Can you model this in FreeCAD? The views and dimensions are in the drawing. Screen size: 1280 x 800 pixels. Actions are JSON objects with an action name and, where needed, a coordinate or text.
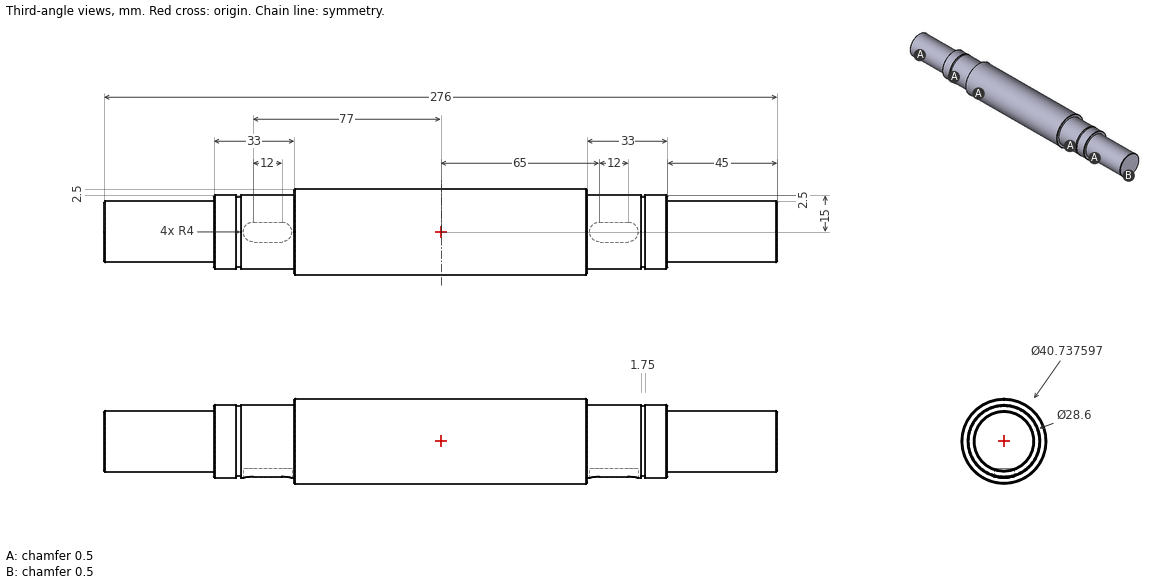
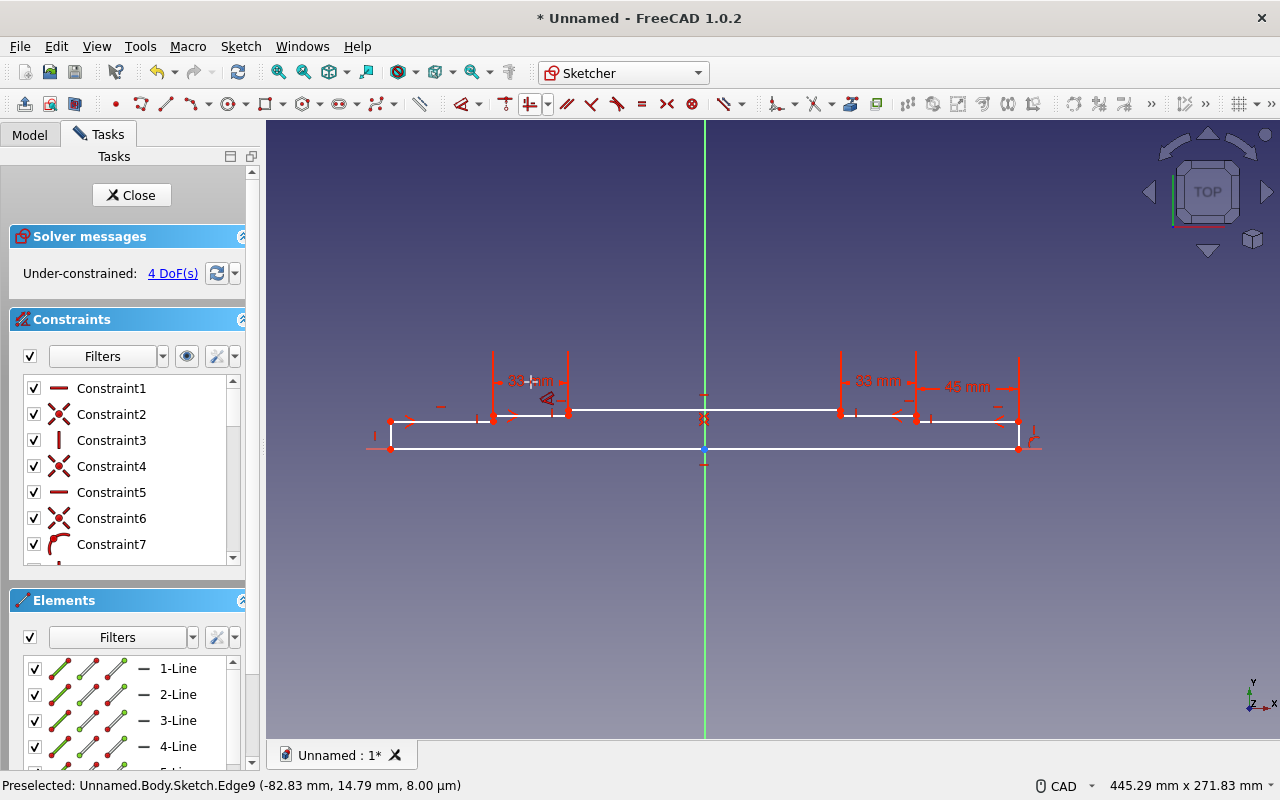
{"action": "scroll", "coordinate": [916, 419], "scroll_direction": "up", "scroll_amount": 10}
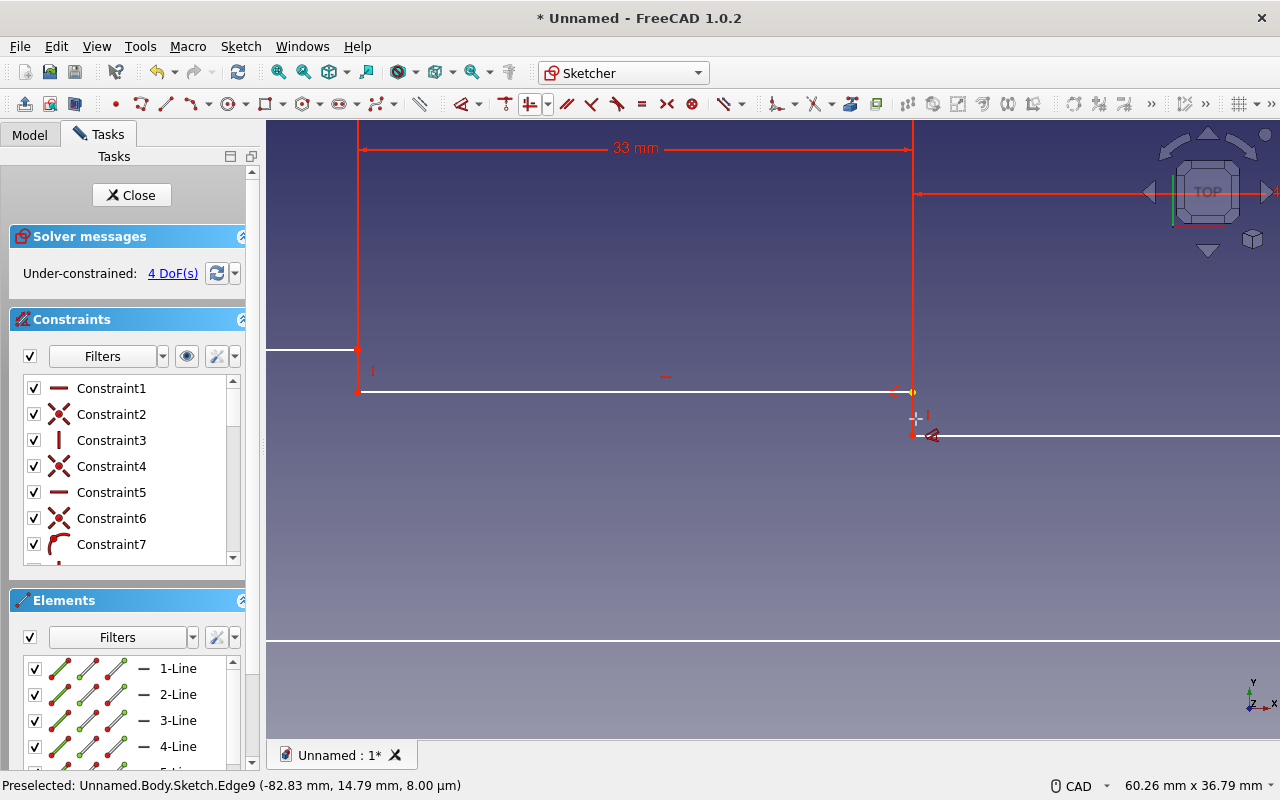
{"action": "left_click", "coordinate": [913, 414]}
{"action": "left_click", "coordinate": [947, 414]}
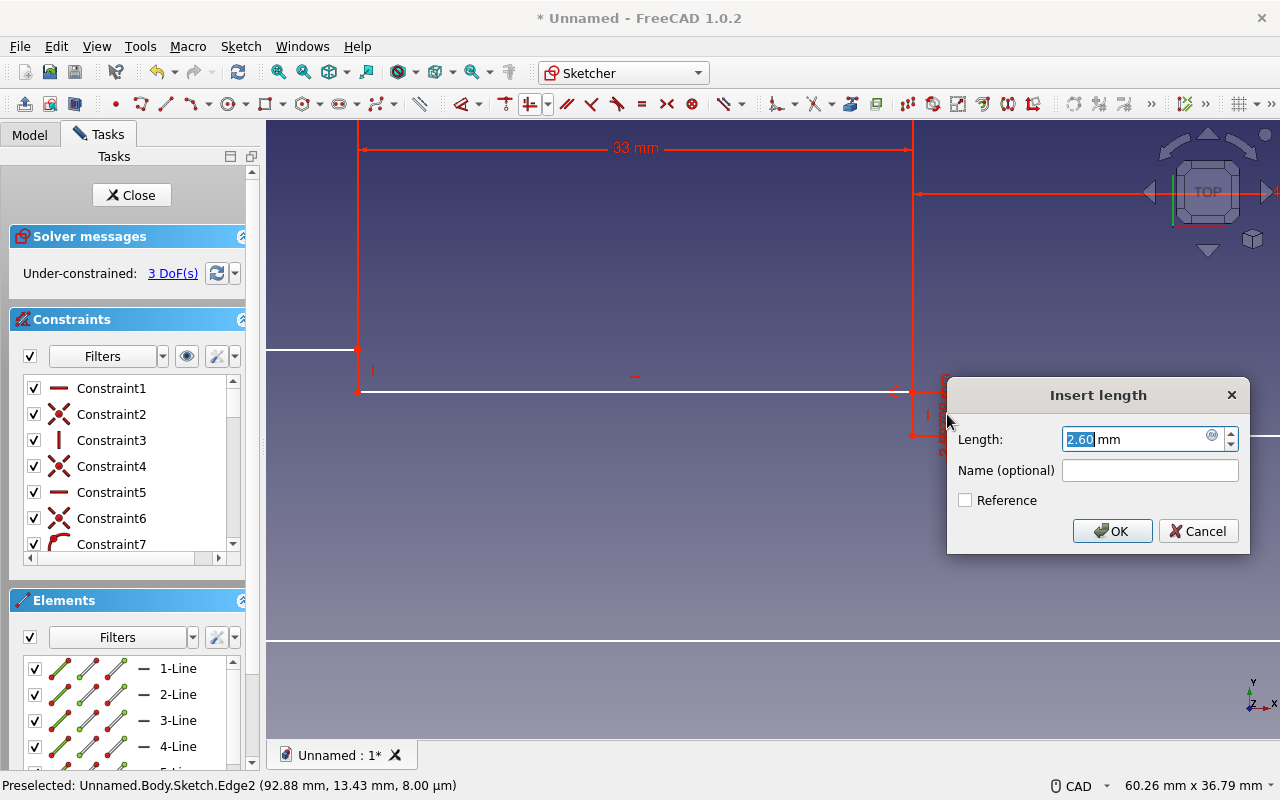
{"action": "type", "text": "2.5"}
{"action": "key", "text": "Return"}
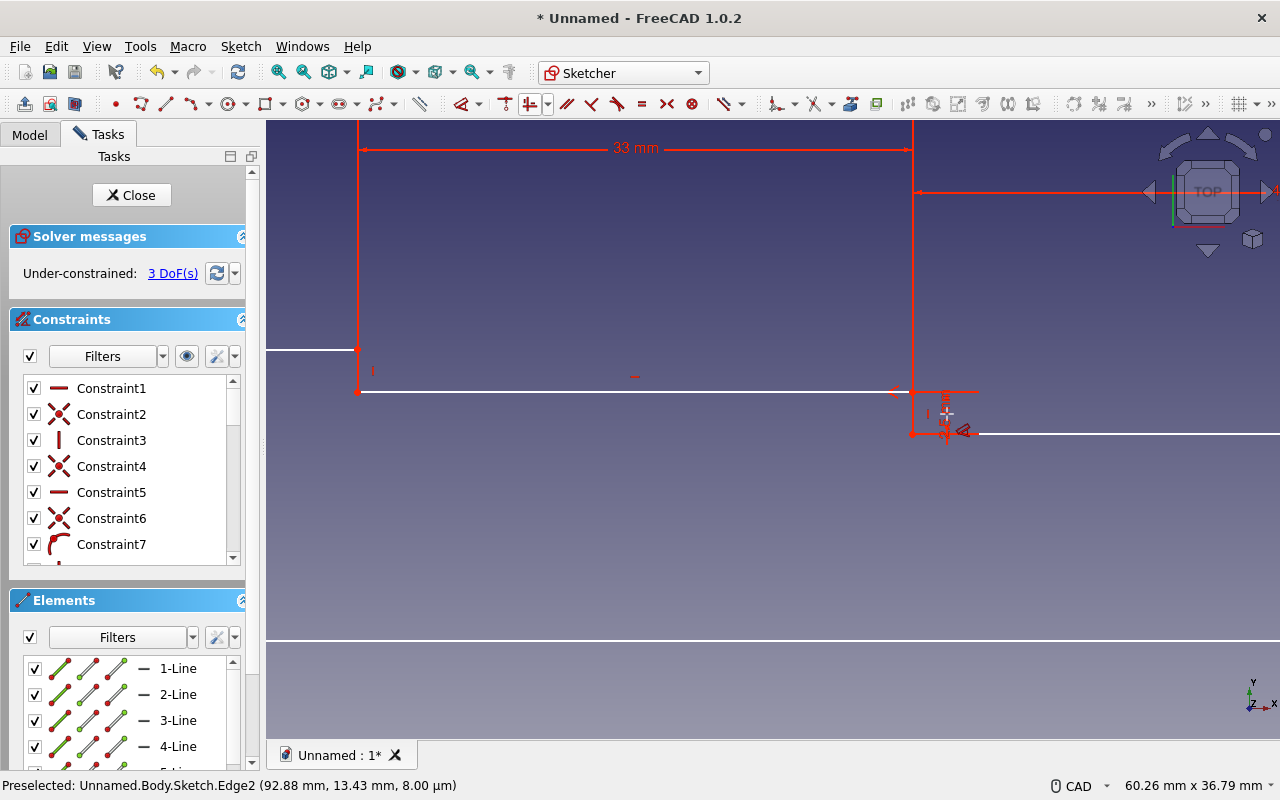
{"action": "scroll", "coordinate": [916, 419], "scroll_direction": "down", "scroll_amount": 10}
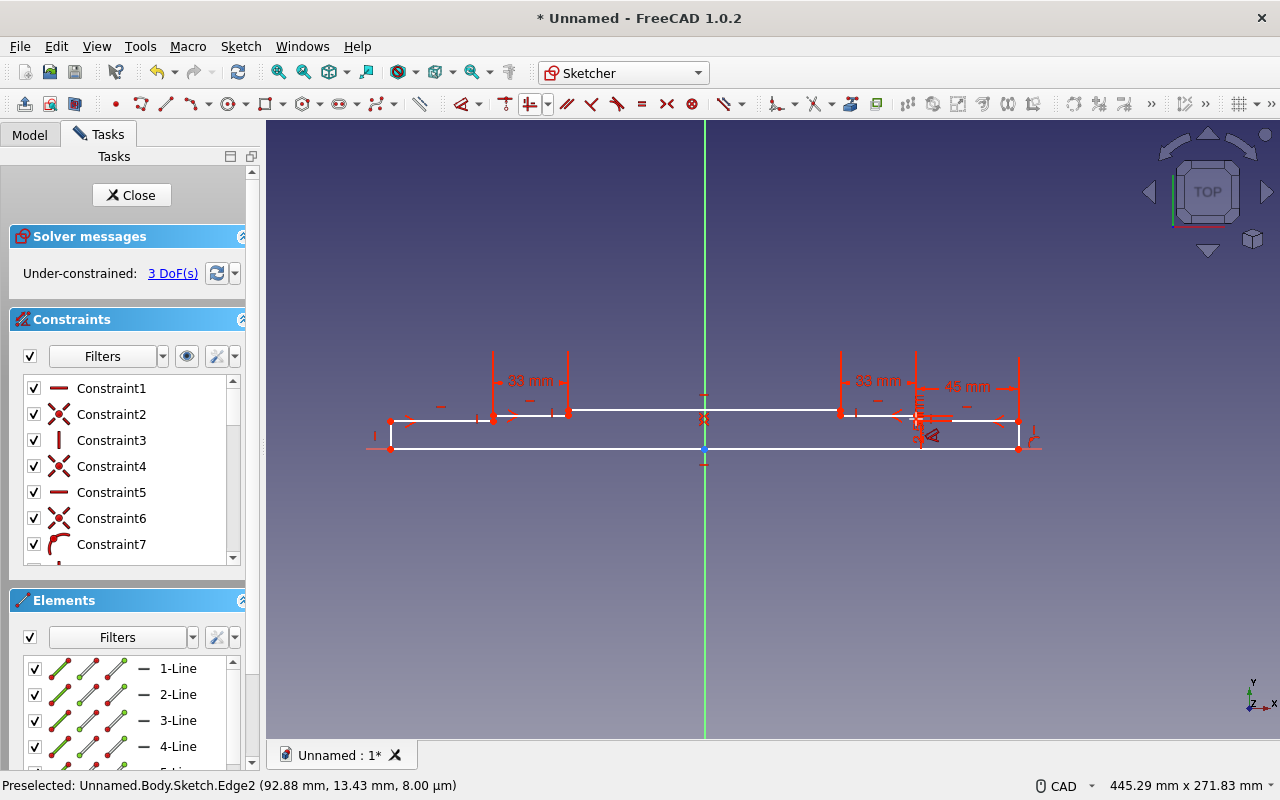
{"action": "left_click", "coordinate": [893, 449]}
{"action": "left_click", "coordinate": [560, 483]}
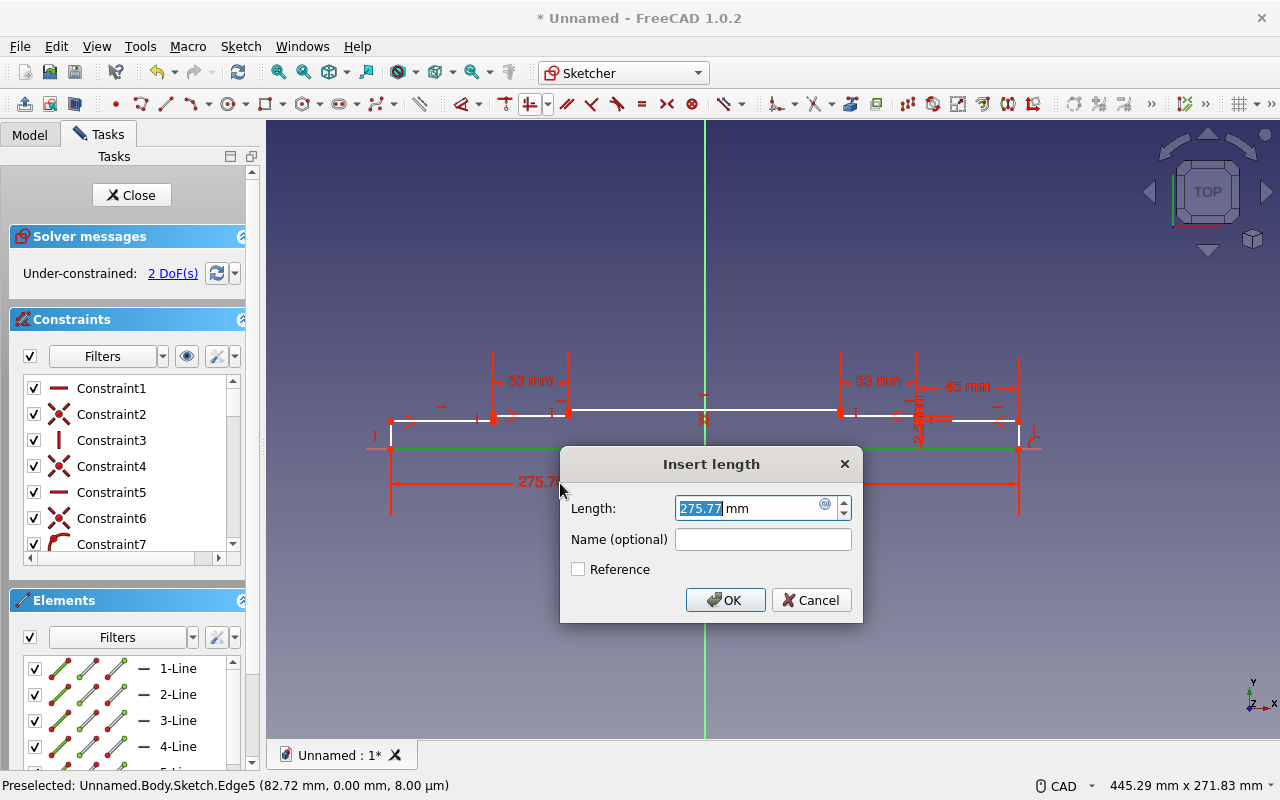
{"action": "type", "text": "276"}
{"action": "key", "text": "Return"}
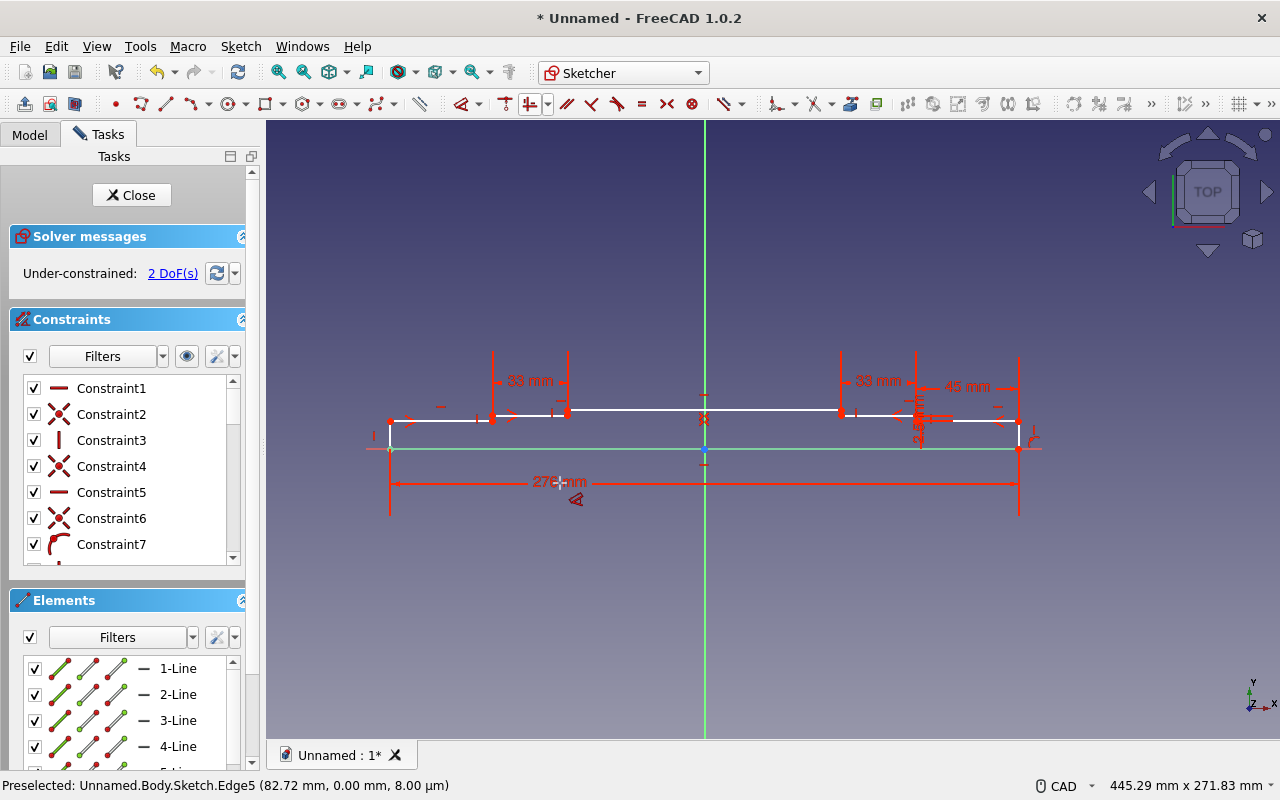
{"action": "scroll", "coordinate": [568, 413], "scroll_direction": "up", "scroll_amount": 10}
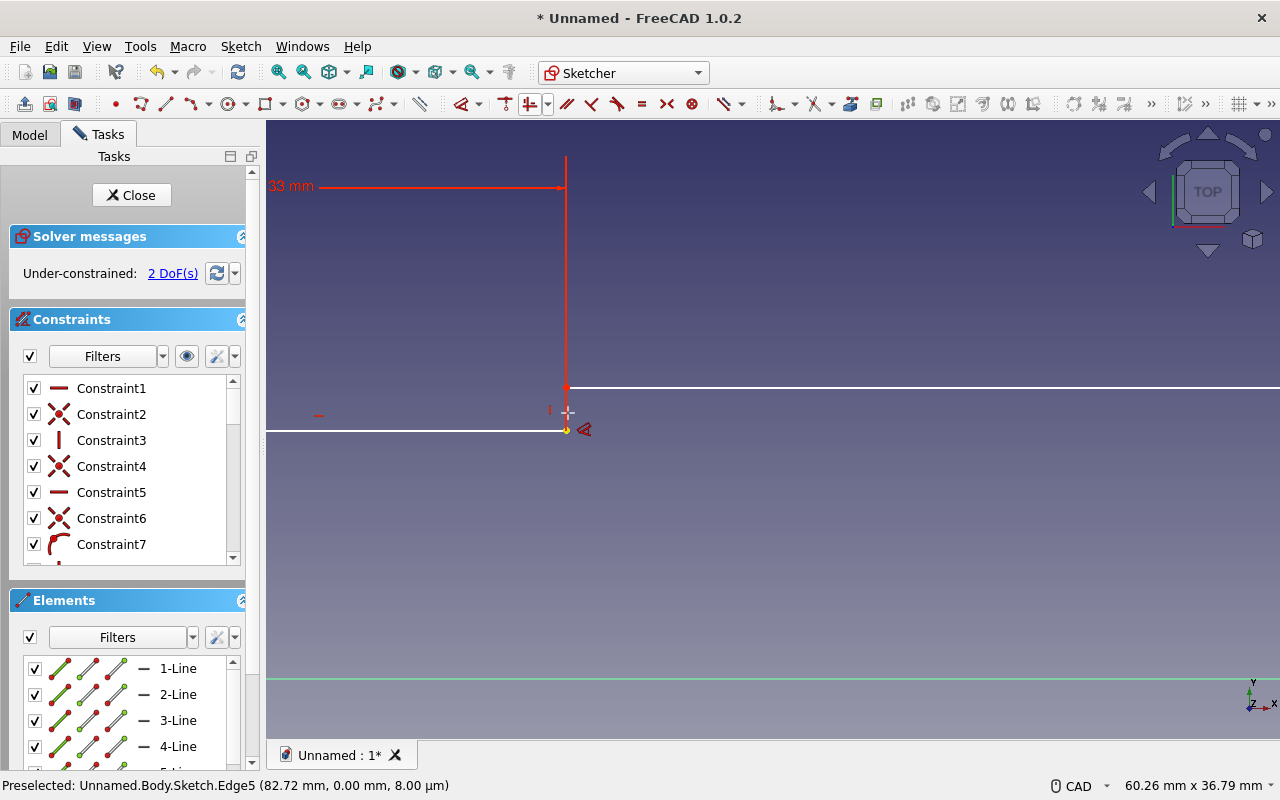
{"action": "left_click", "coordinate": [566, 409]}
{"action": "left_click", "coordinate": [532, 409]}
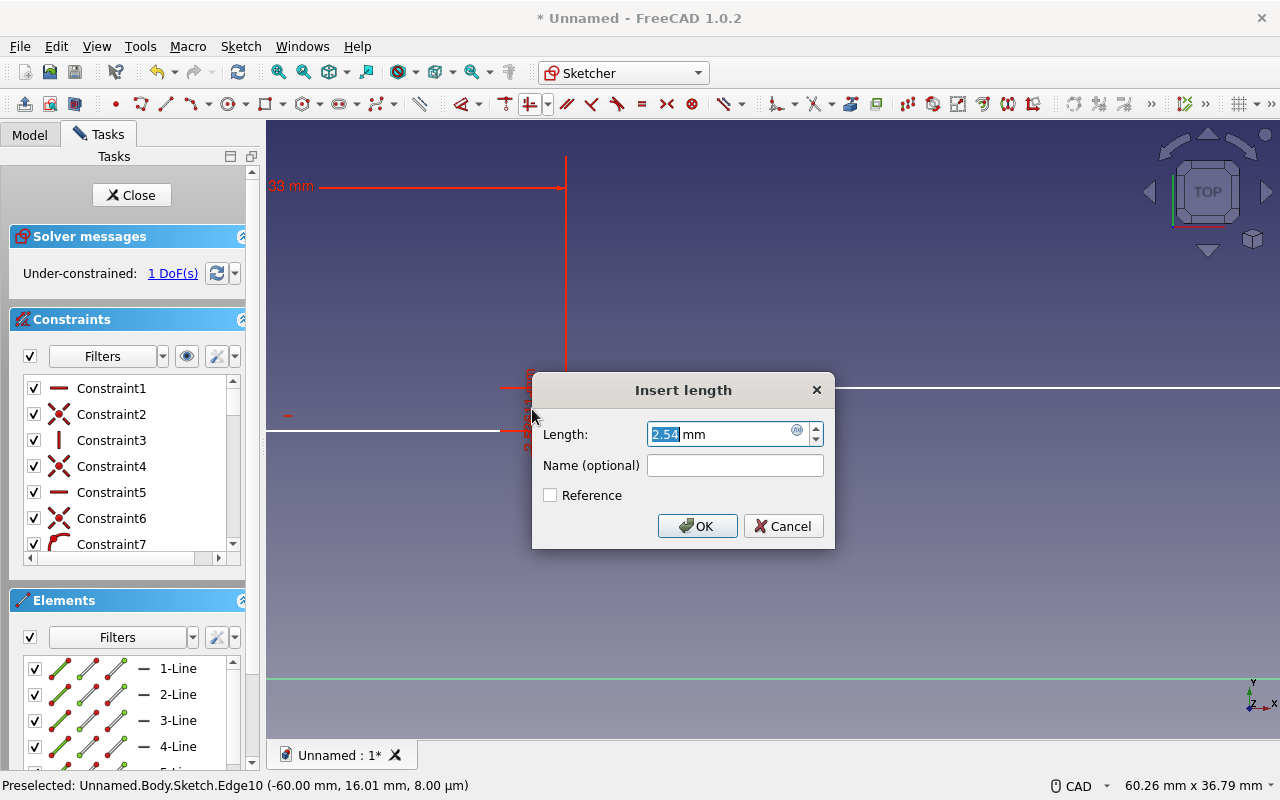
{"action": "type", "text": "2.5"}
{"action": "key", "text": "Return"}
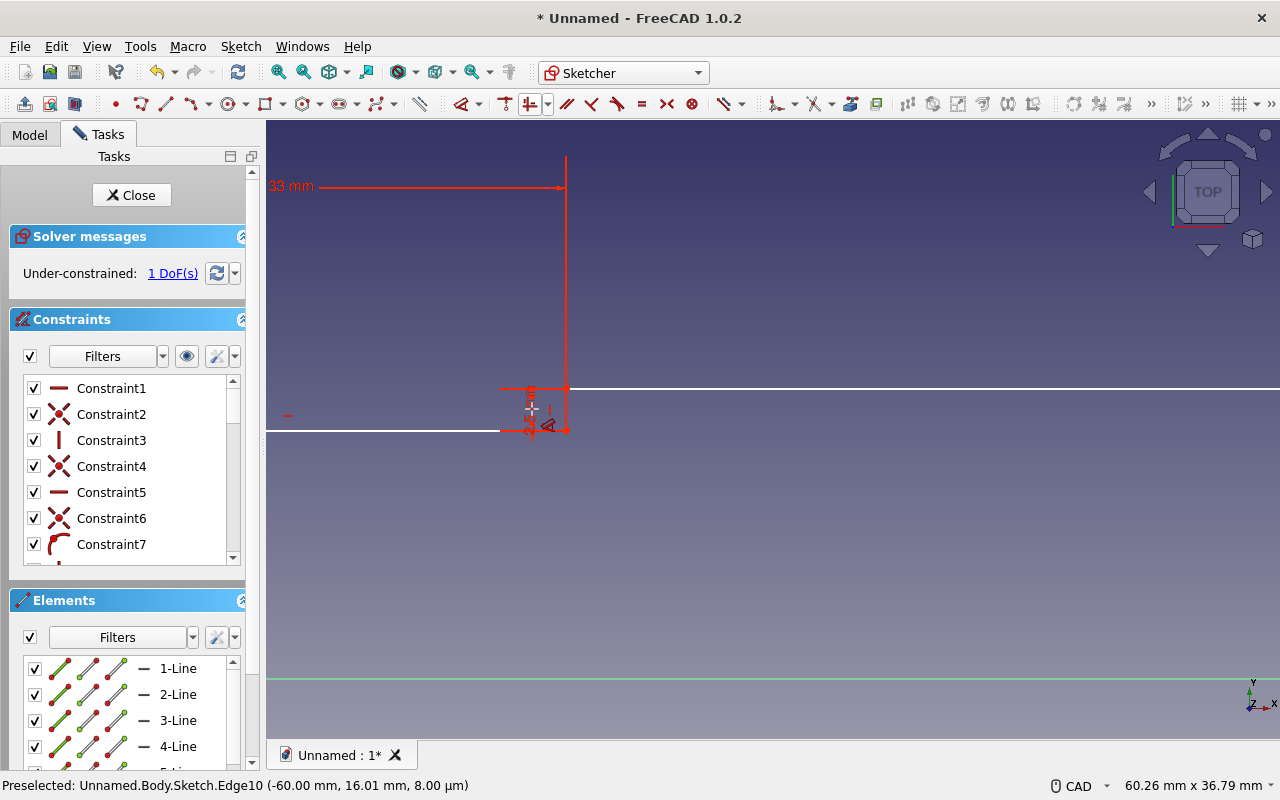
{"action": "scroll", "coordinate": [568, 413], "scroll_direction": "down", "scroll_amount": 10}